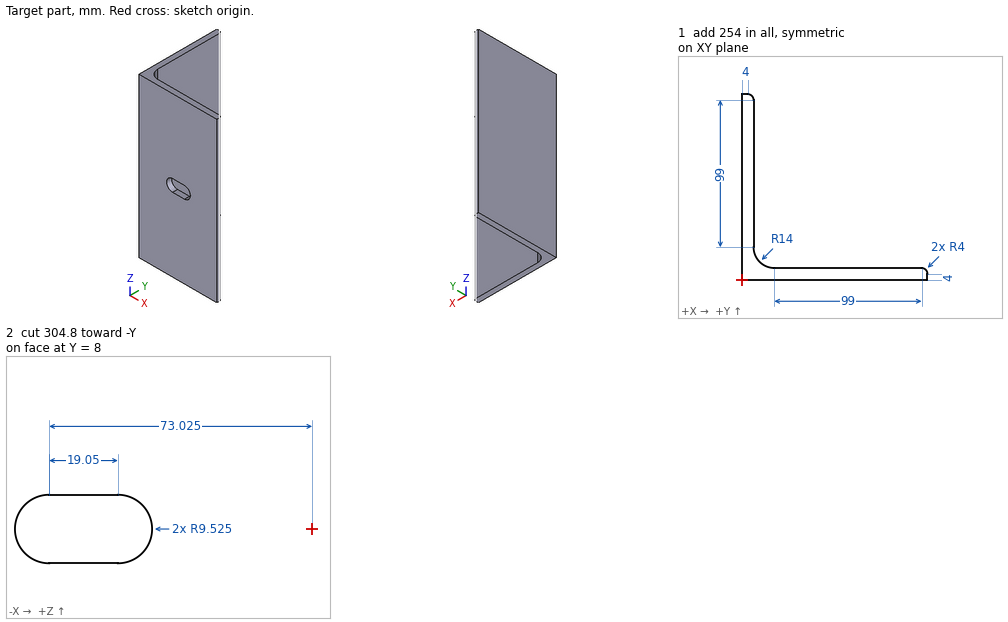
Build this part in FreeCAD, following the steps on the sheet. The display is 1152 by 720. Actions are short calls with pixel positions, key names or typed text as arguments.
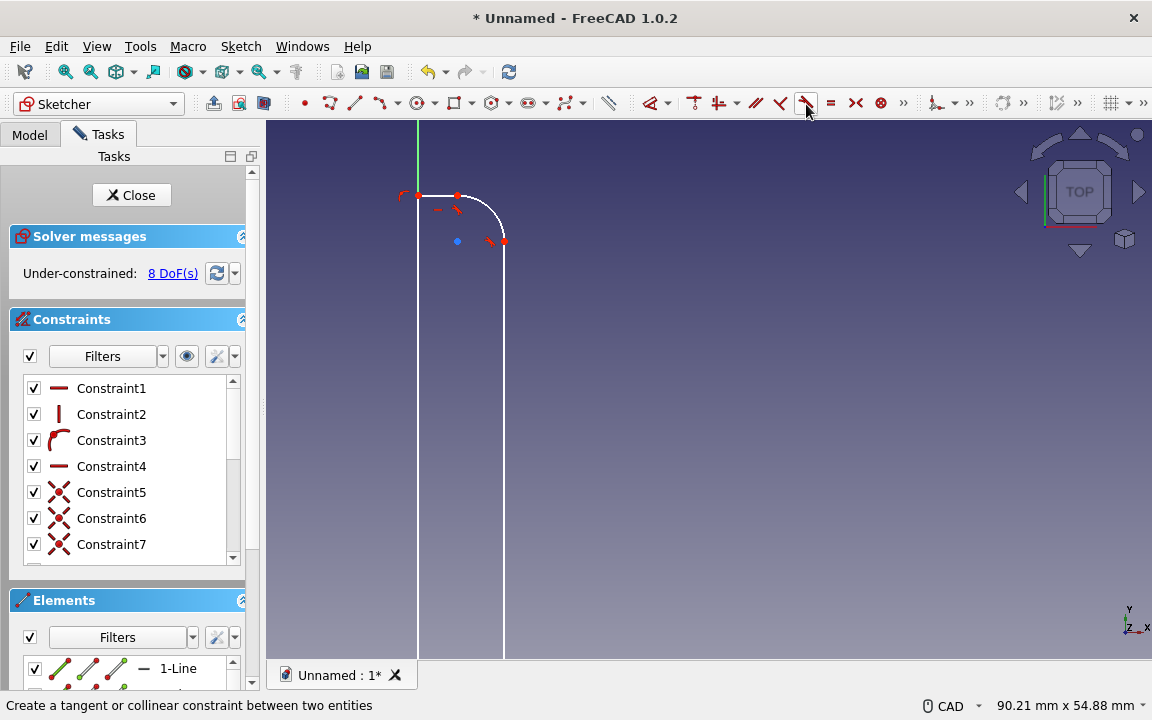
scroll(472, 208, down, 6)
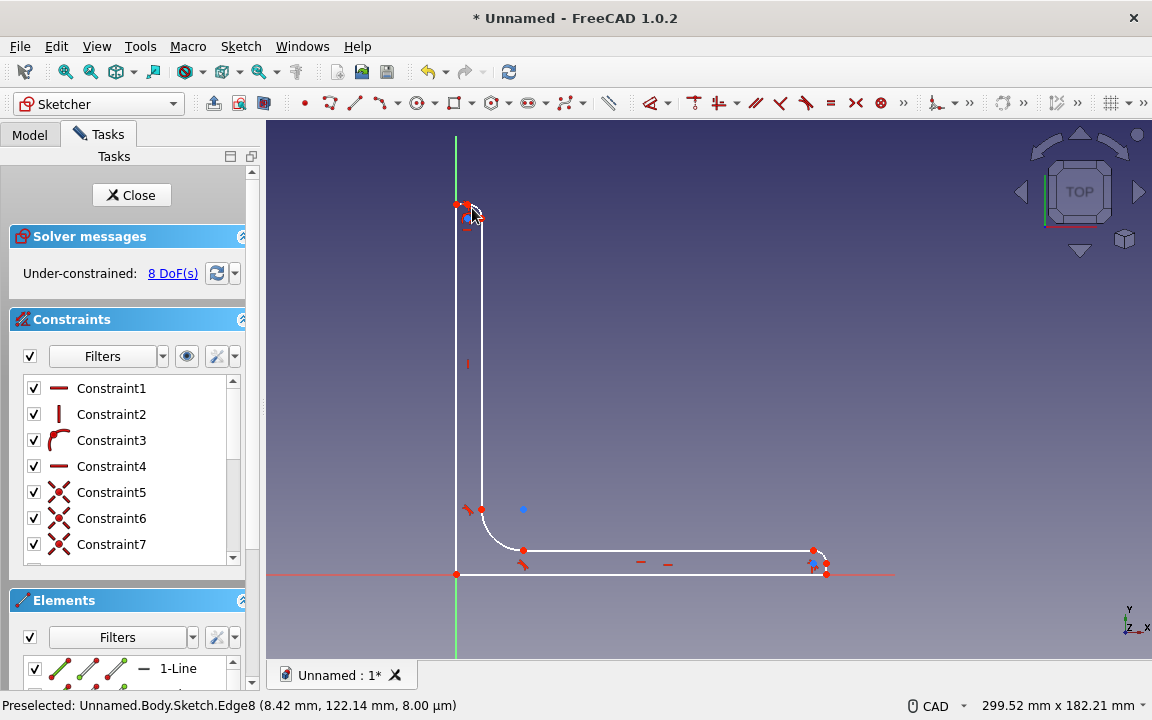
scroll(826, 571, up, 8)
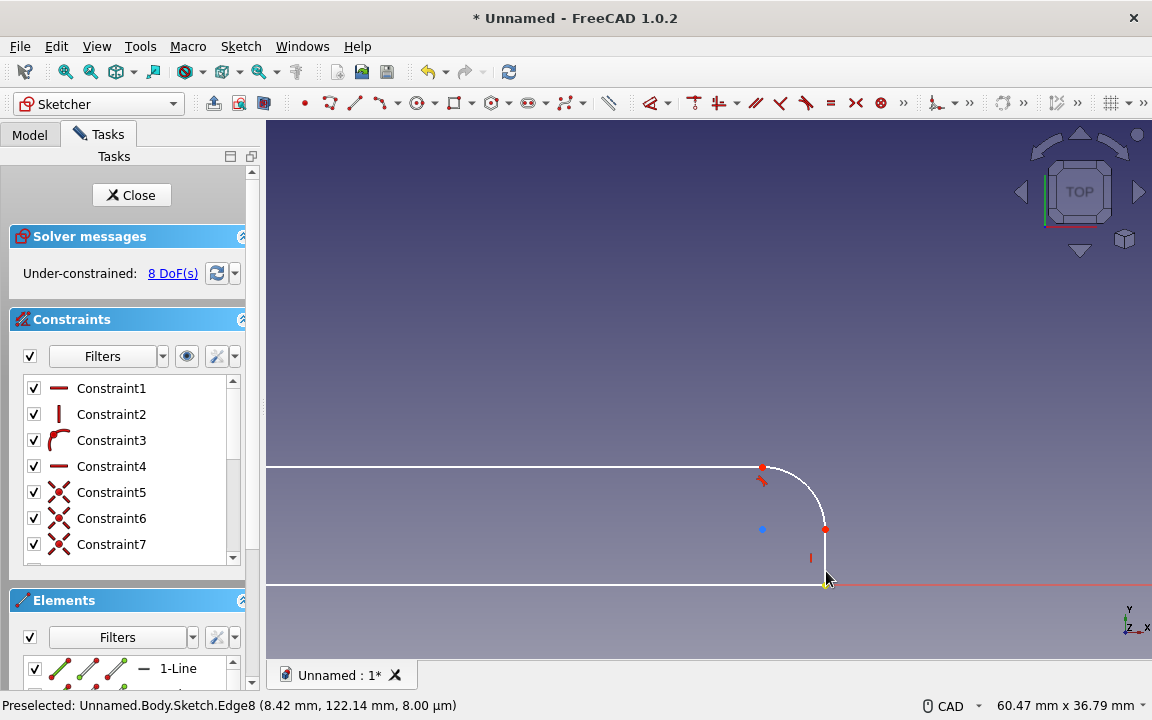
click(825, 568)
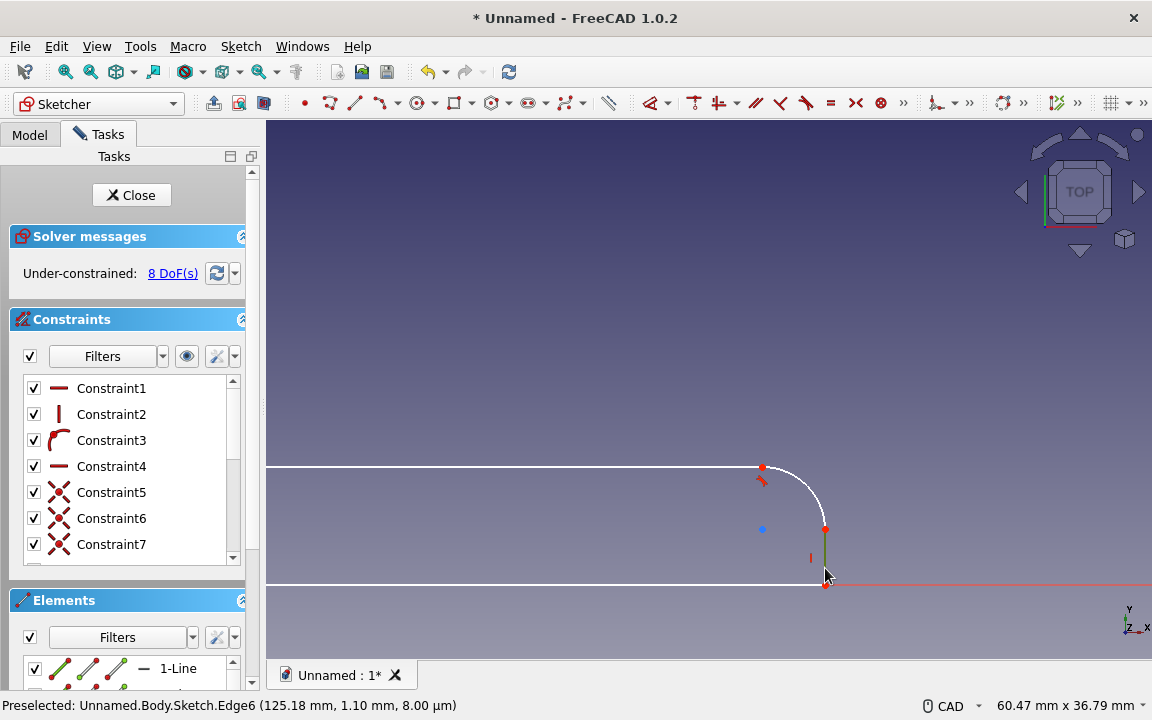
click(818, 501)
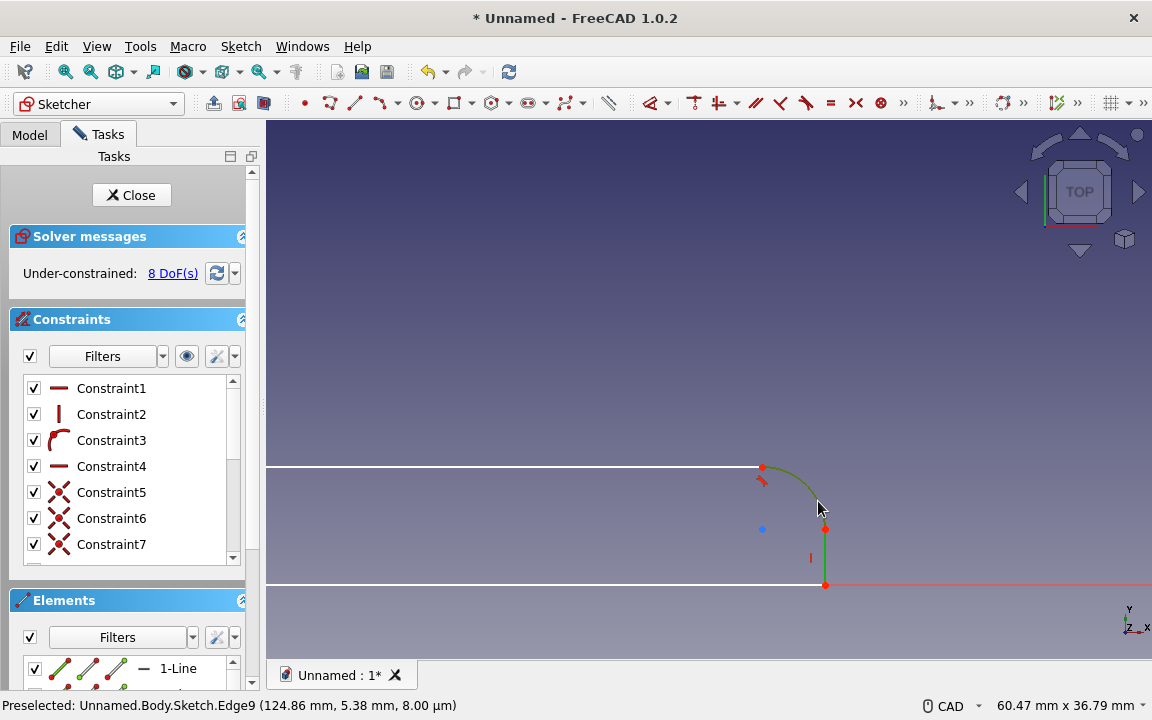
click(806, 104)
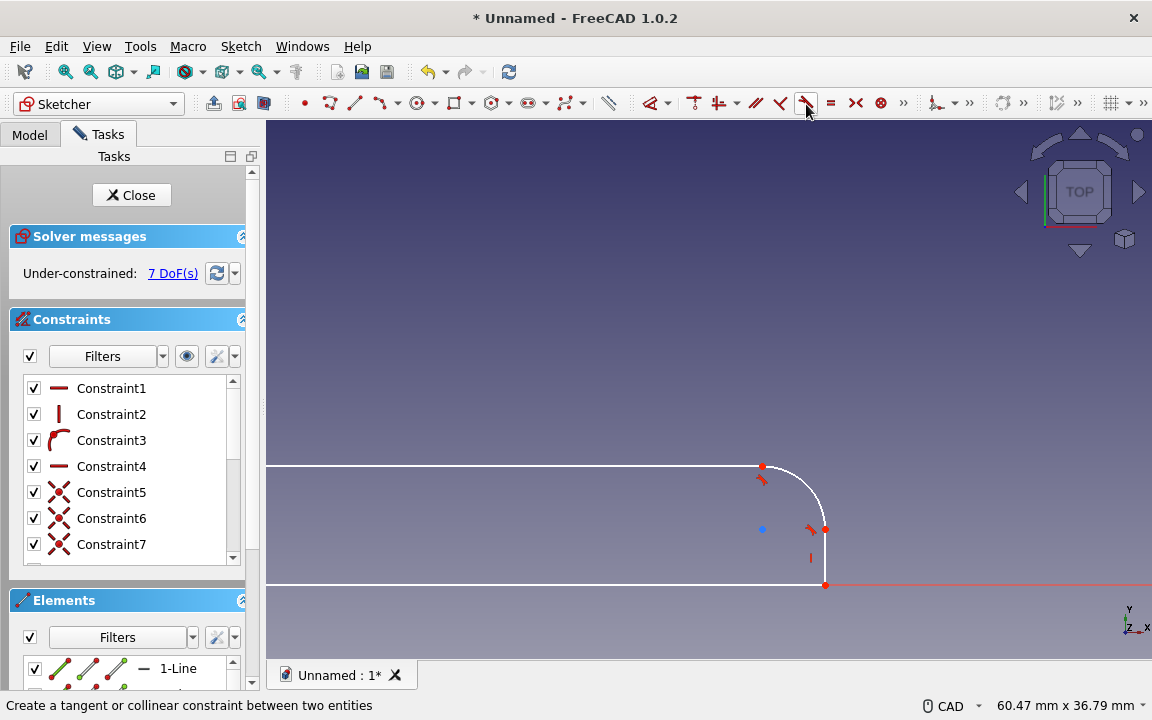
scroll(826, 572, down, 8)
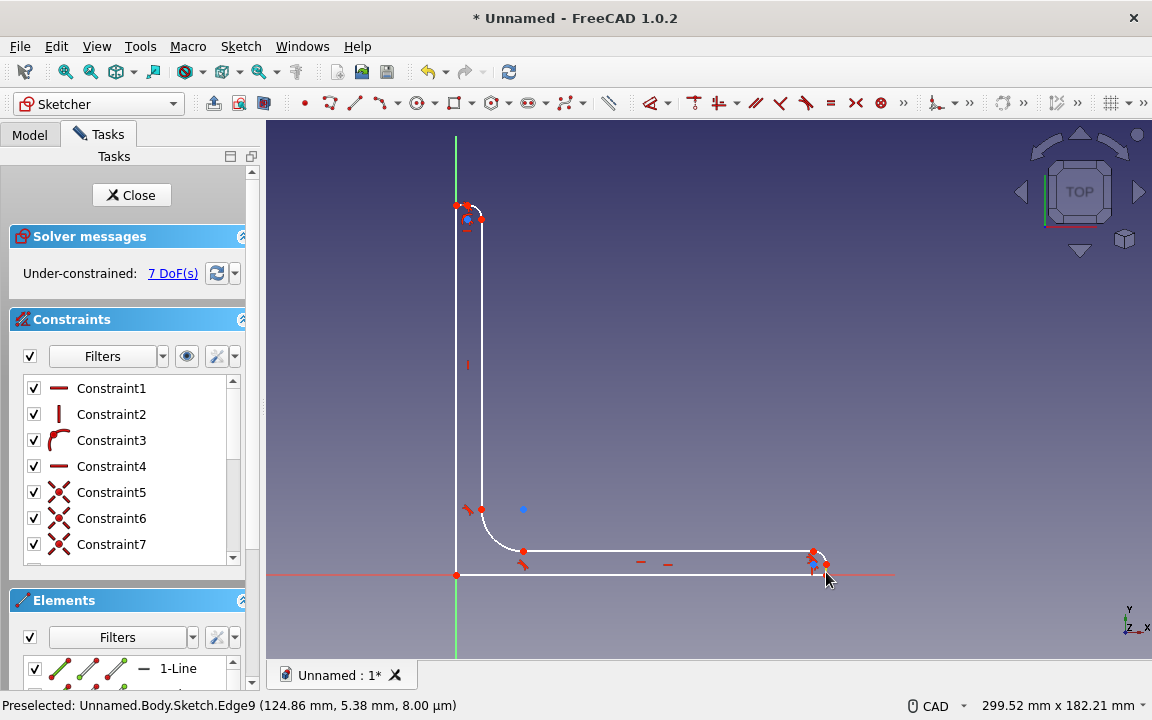
scroll(480, 213, up, 4)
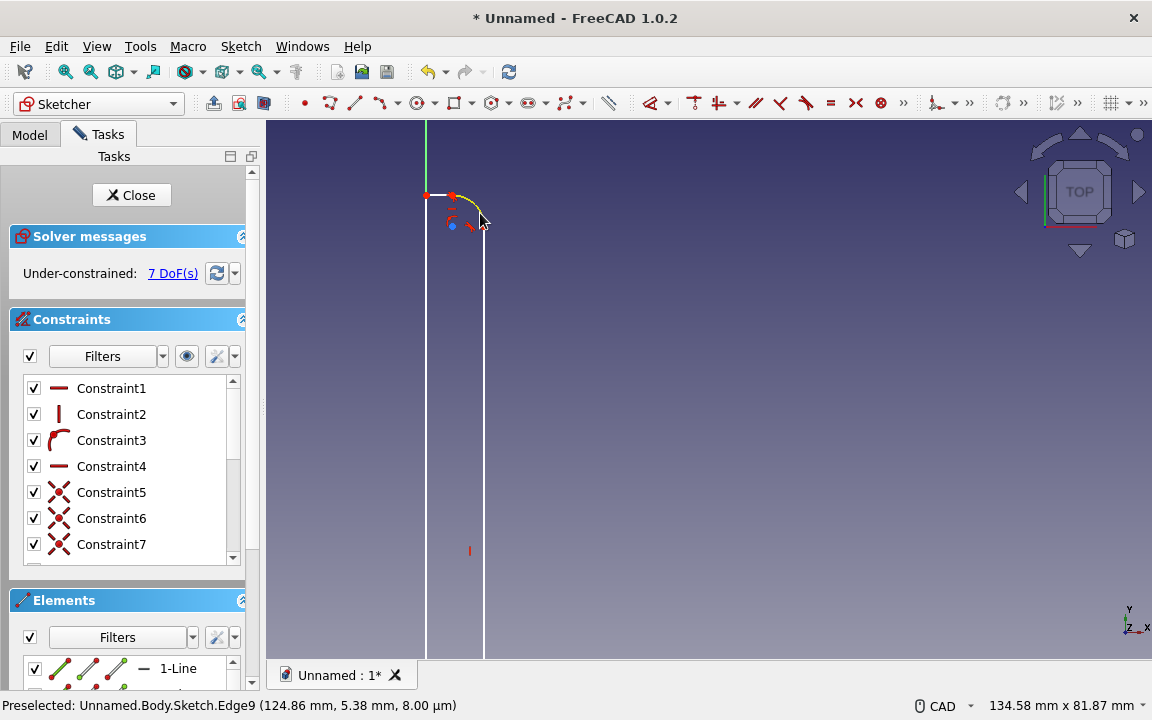
click(481, 212)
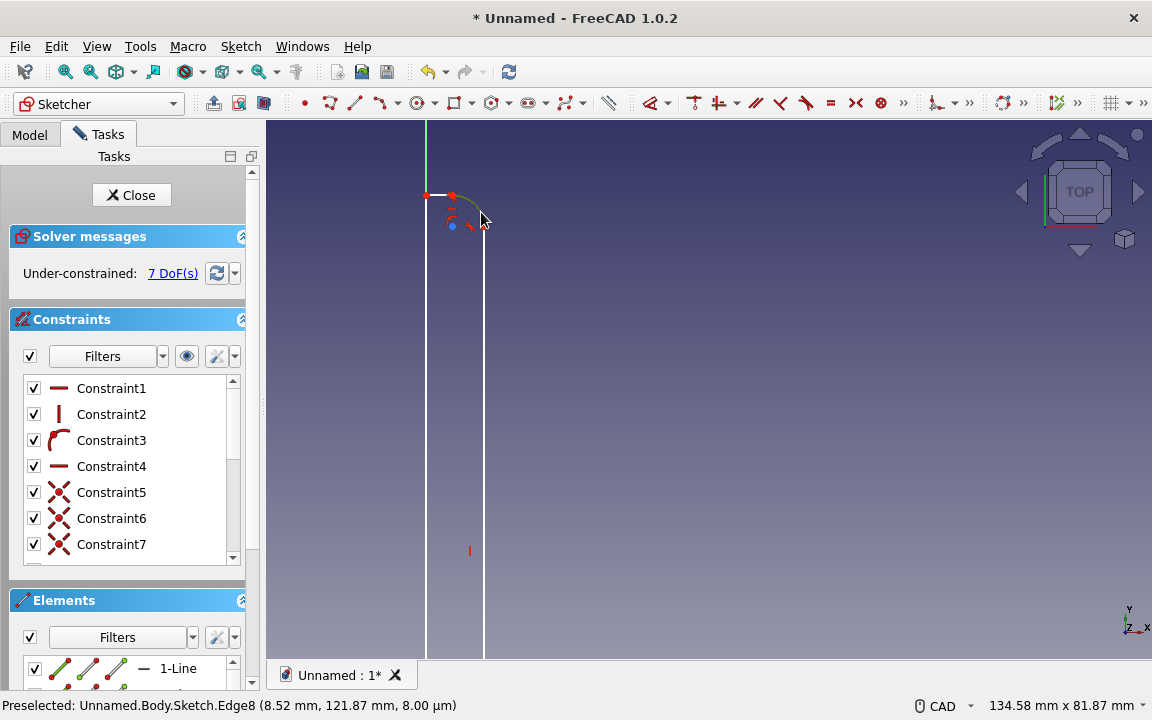
scroll(479, 211, down, 4)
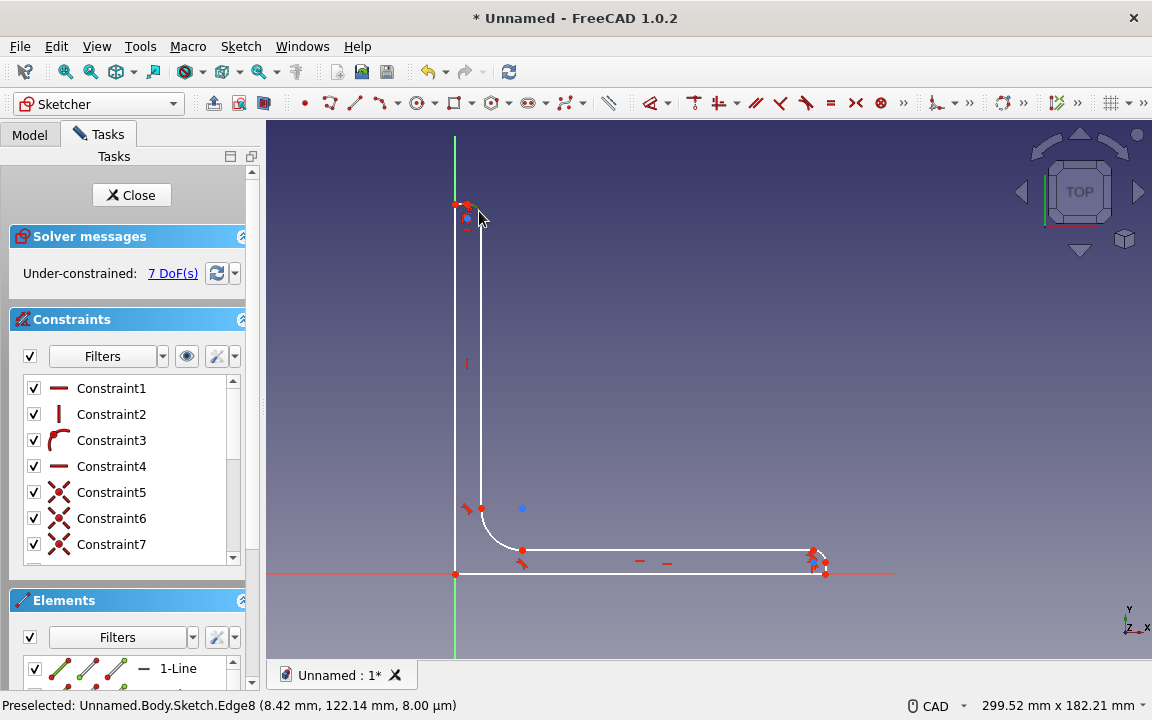
scroll(824, 557, up, 5)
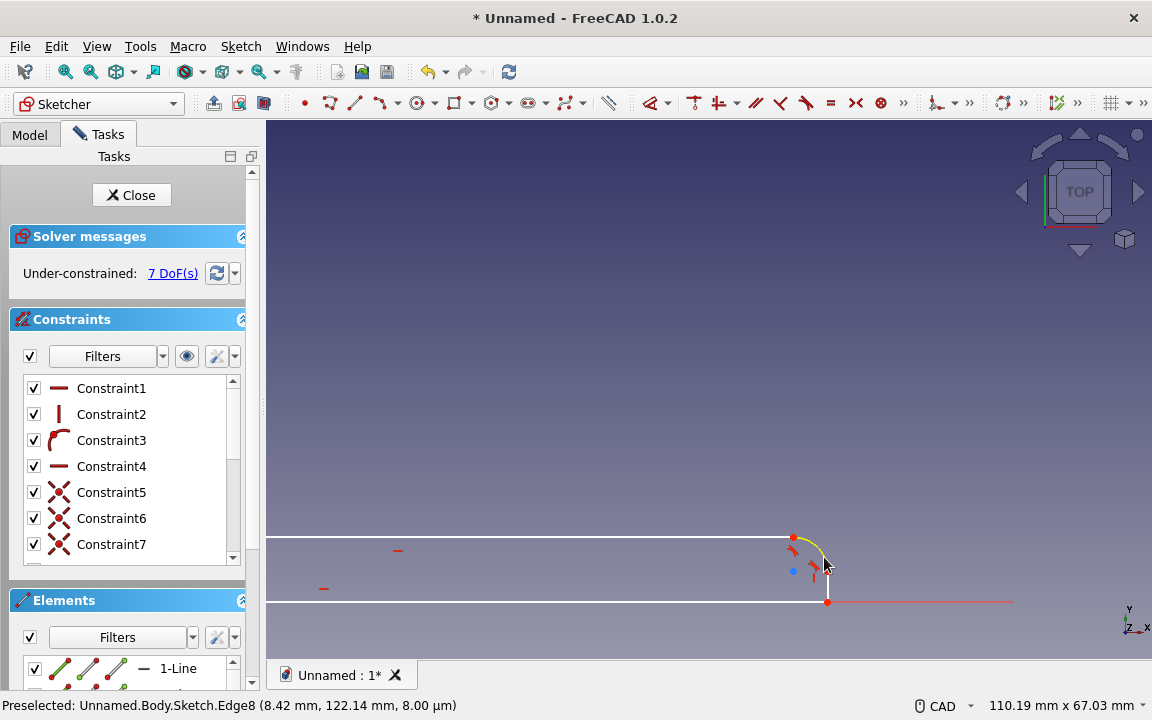
click(824, 556)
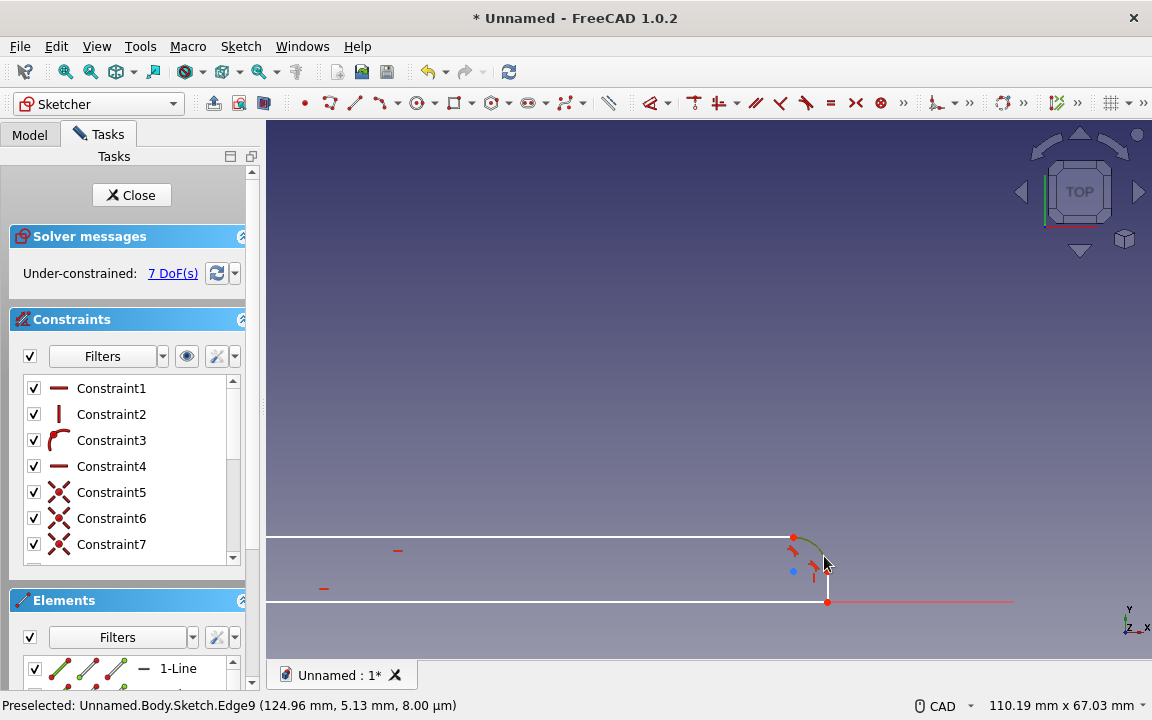
click(831, 104)